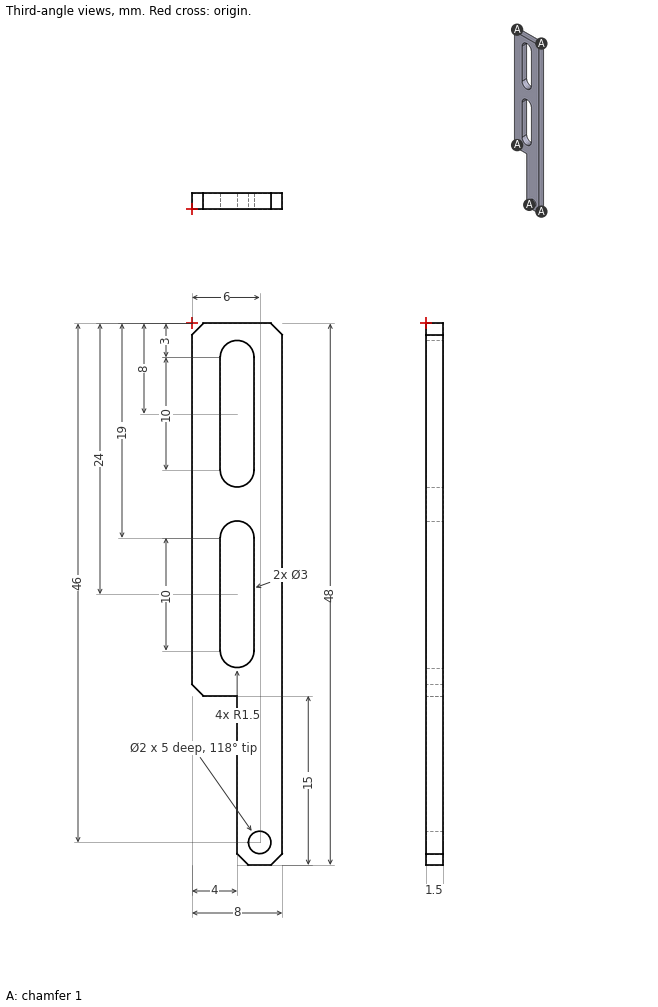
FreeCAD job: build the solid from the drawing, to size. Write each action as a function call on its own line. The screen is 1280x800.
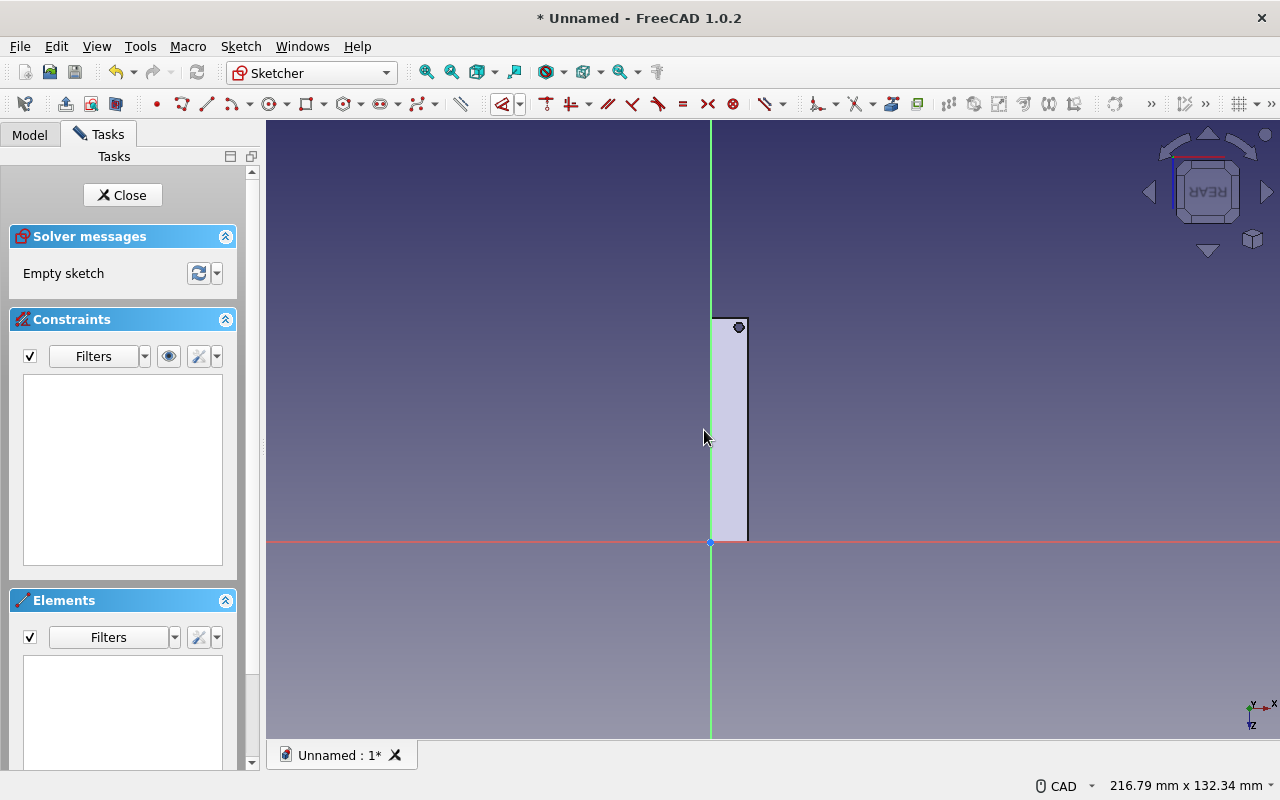
scroll(723, 338, up, 9)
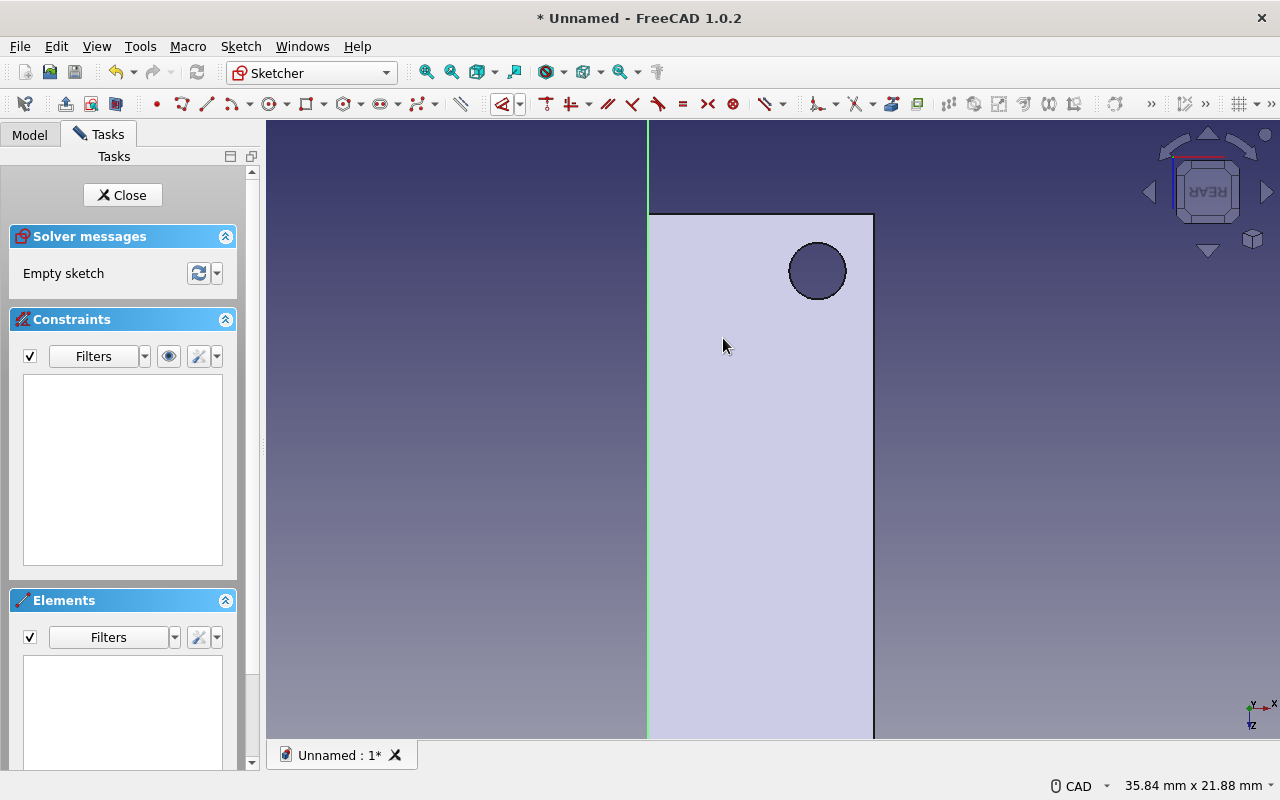
key(g)
key(r)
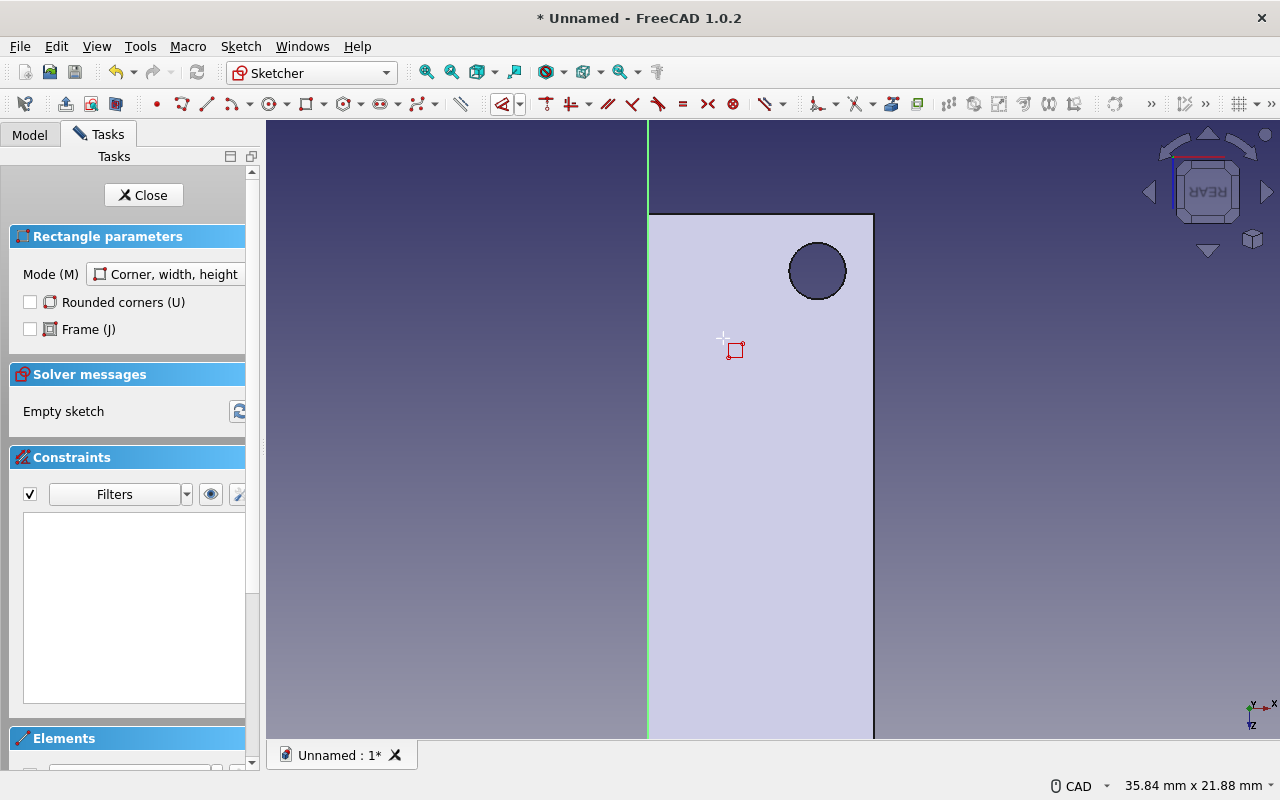
click(648, 214)
move(761, 639)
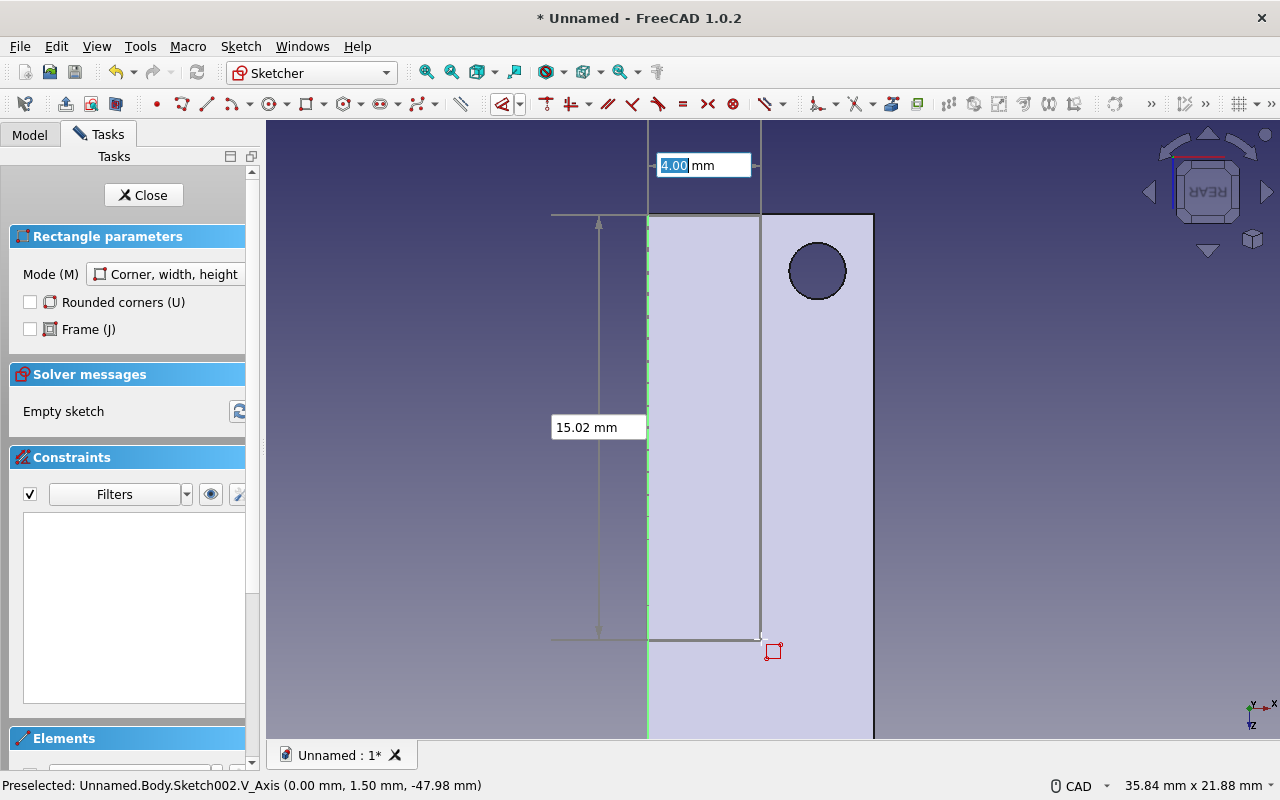
text(4)
key(Tab)
text(15)
key(Return)
key(Escape)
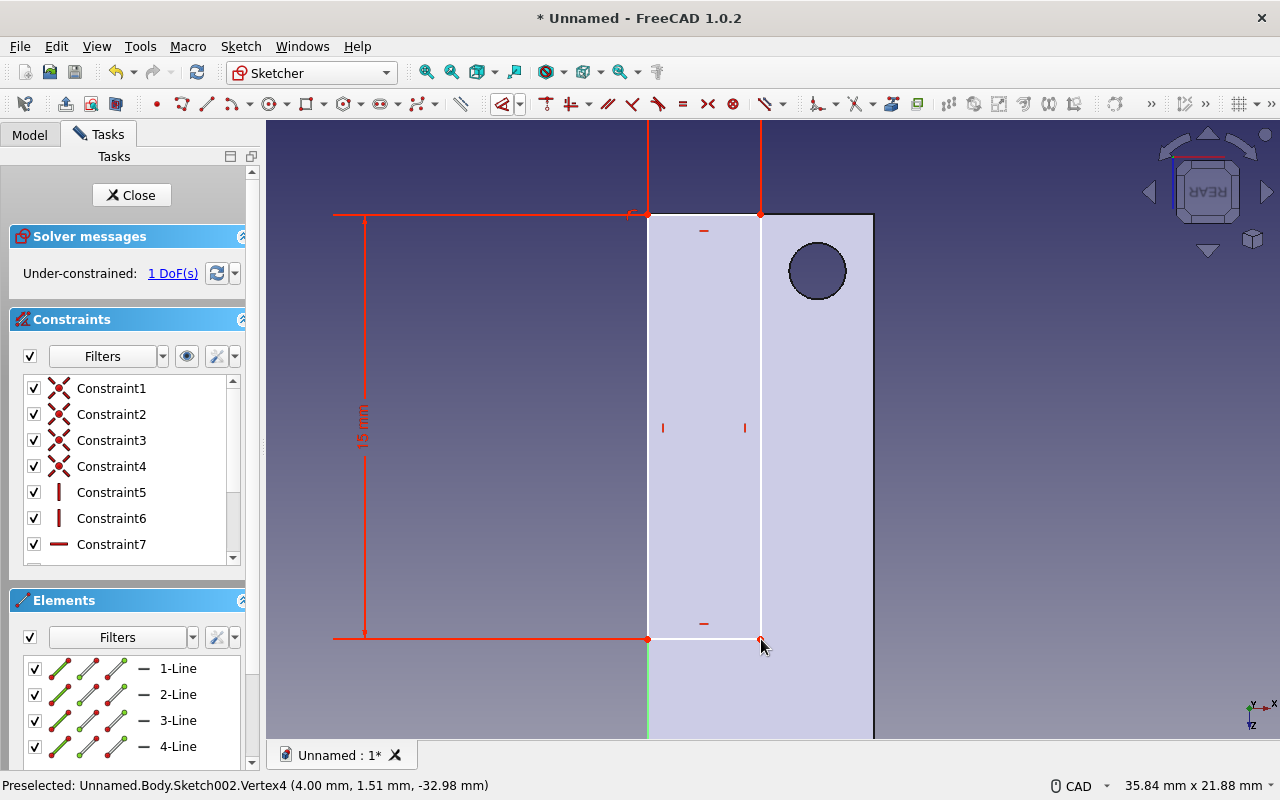
click(648, 215)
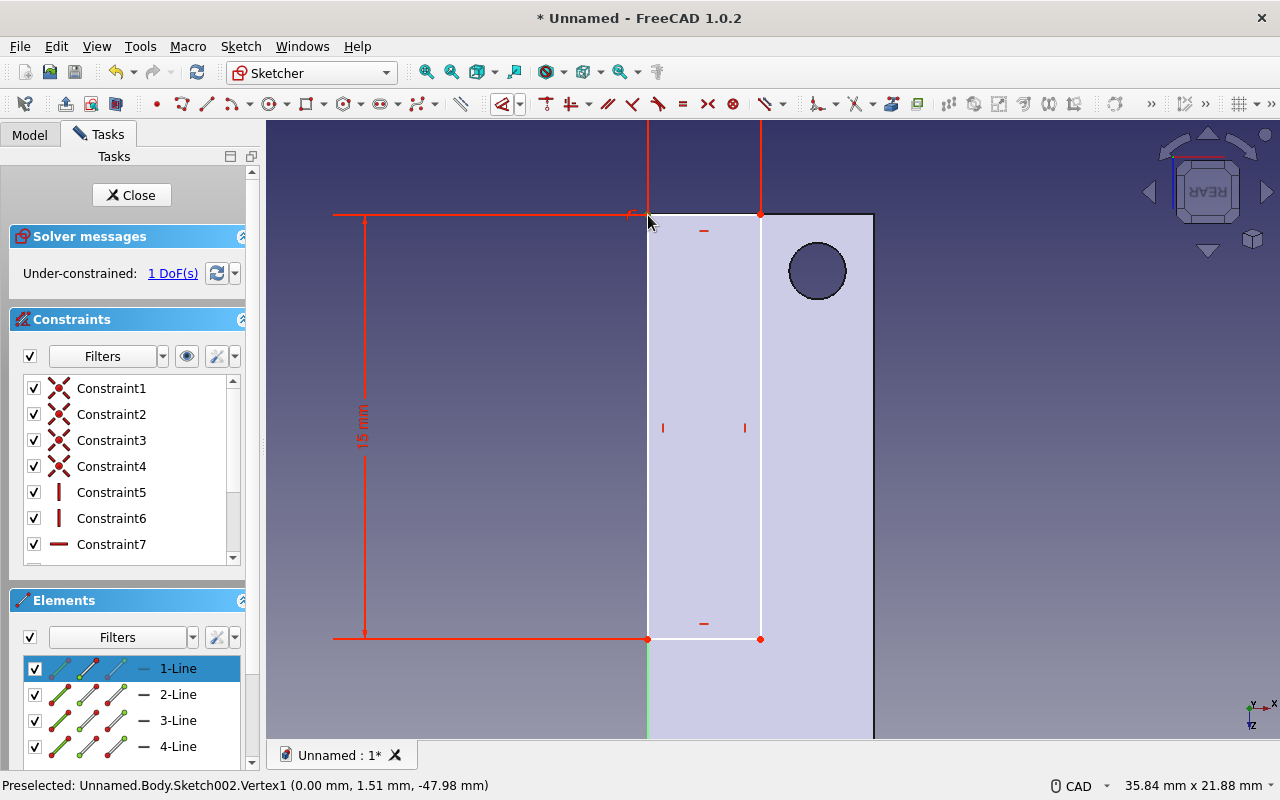
click(520, 104)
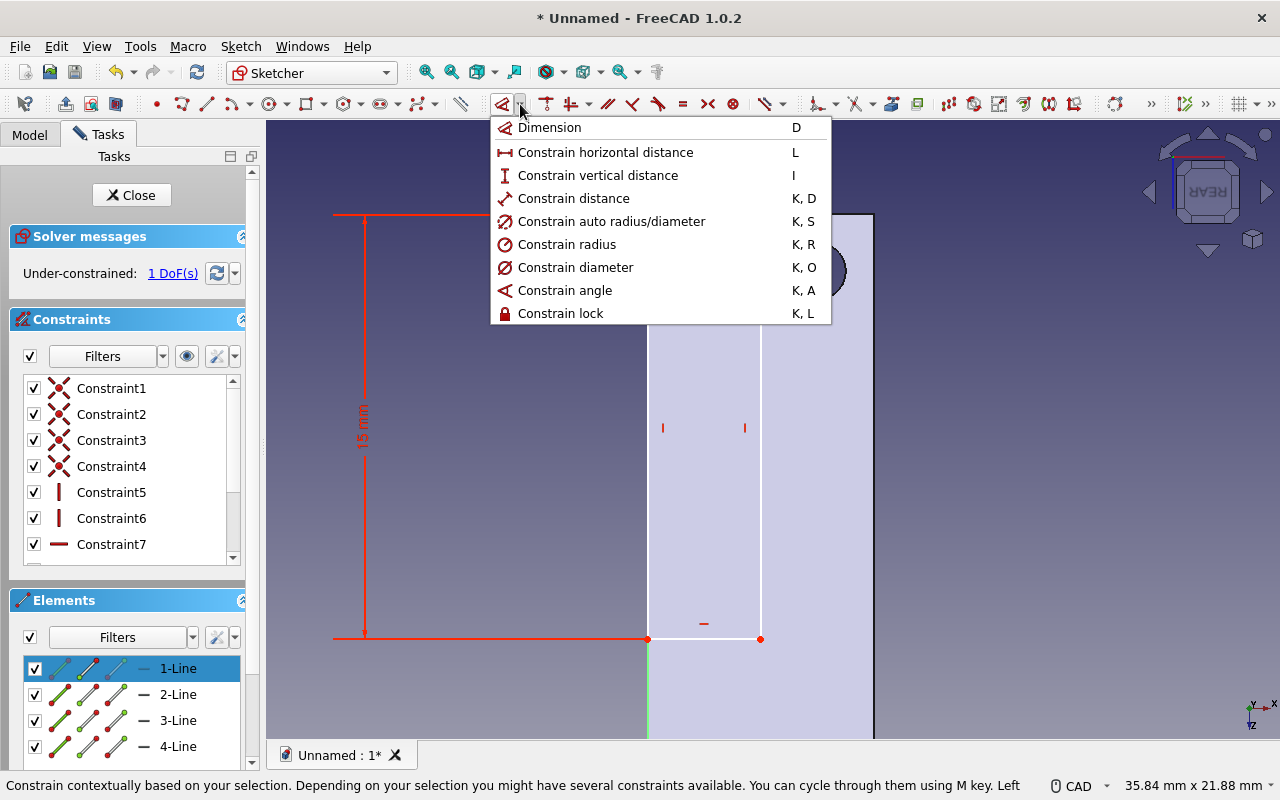
click(661, 176)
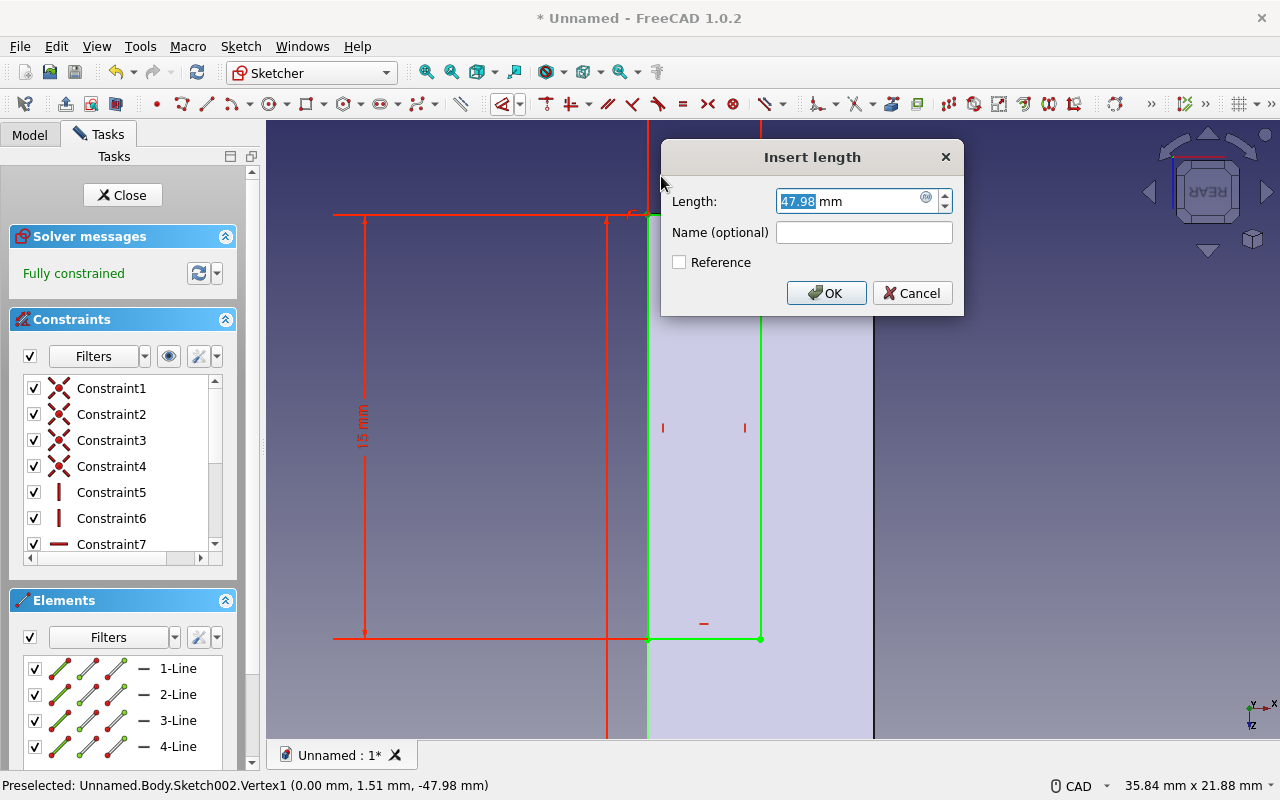
text(48)
key(Return)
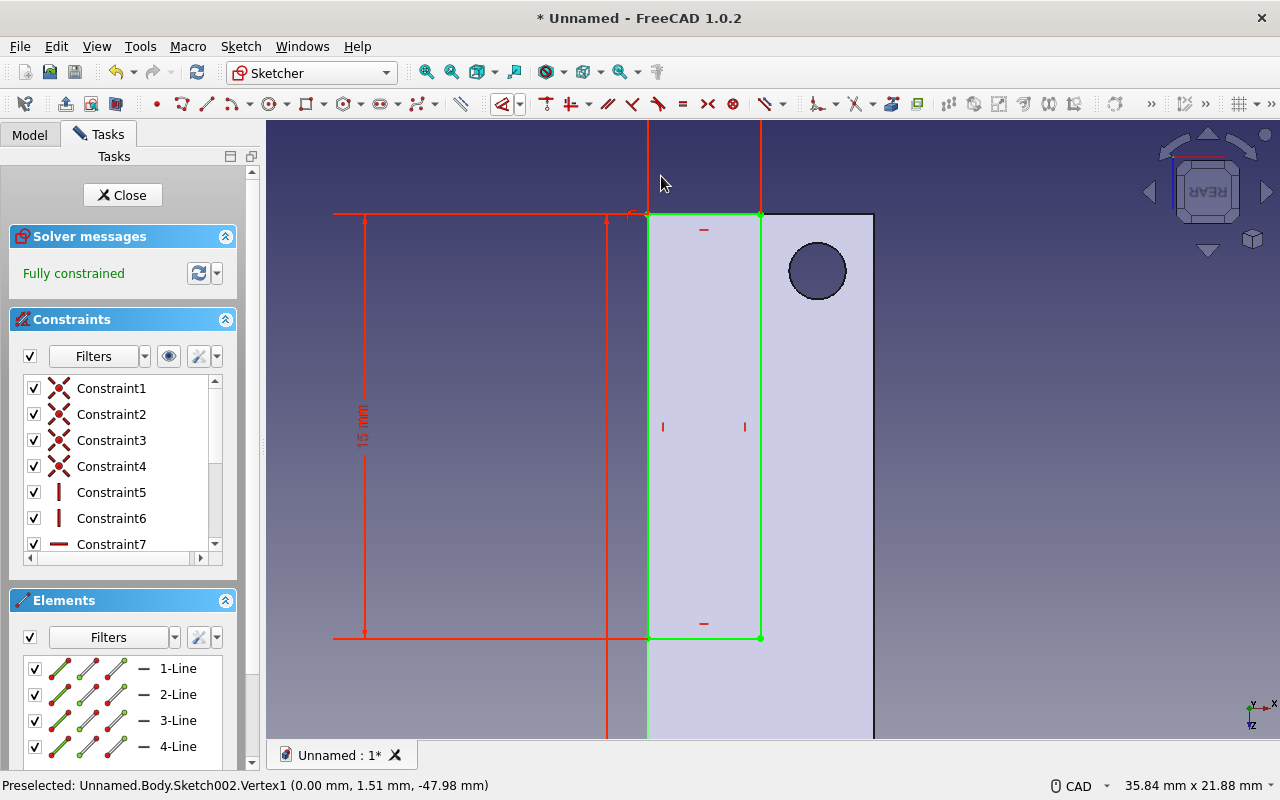
click(123, 195)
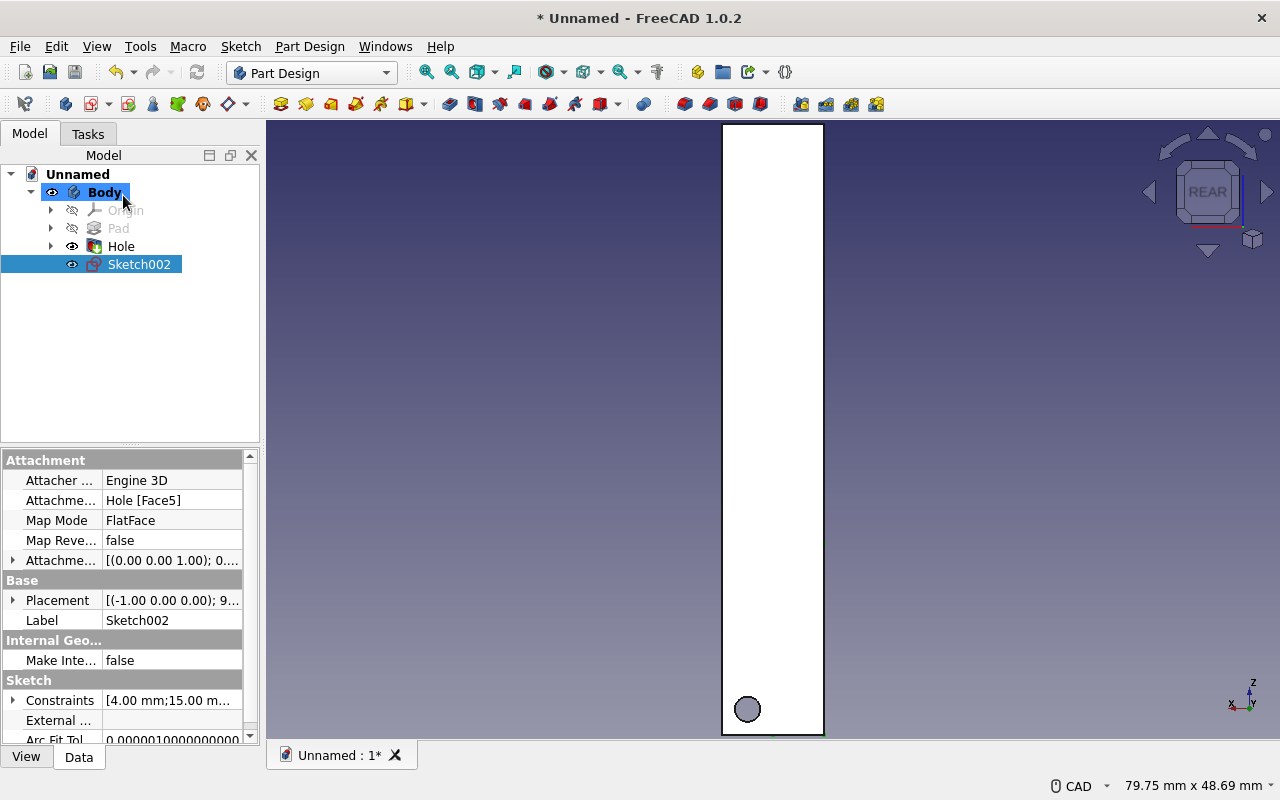
click(450, 104)